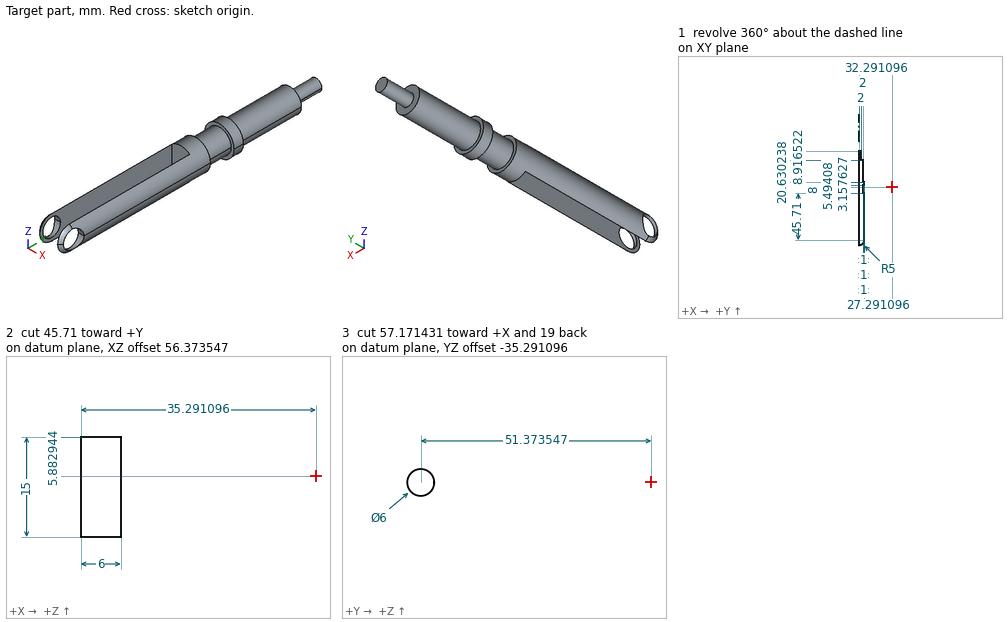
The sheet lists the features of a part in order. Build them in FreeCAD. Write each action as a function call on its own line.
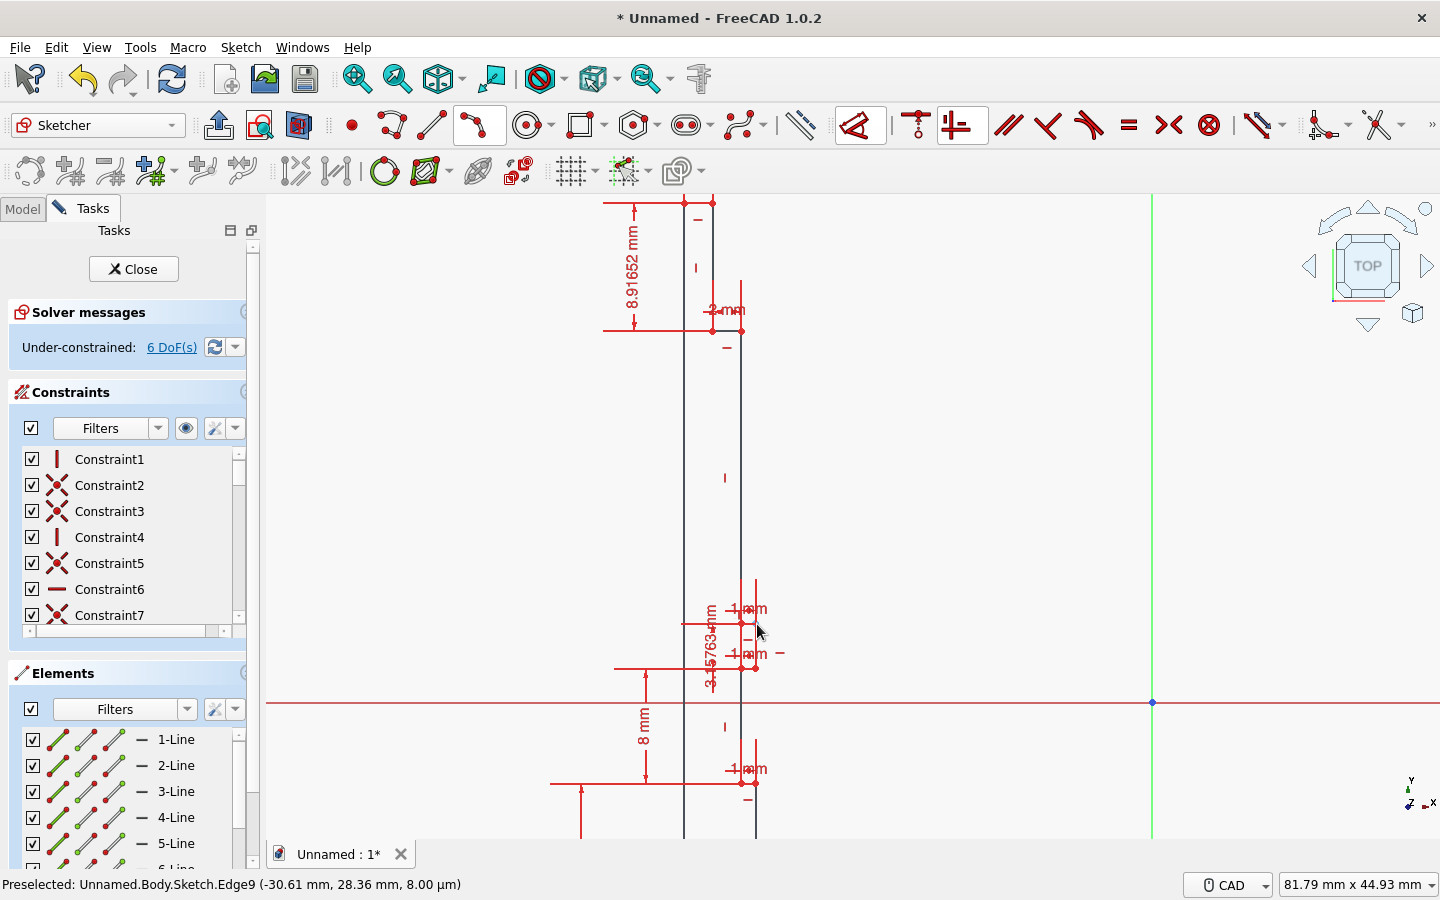
click(756, 624)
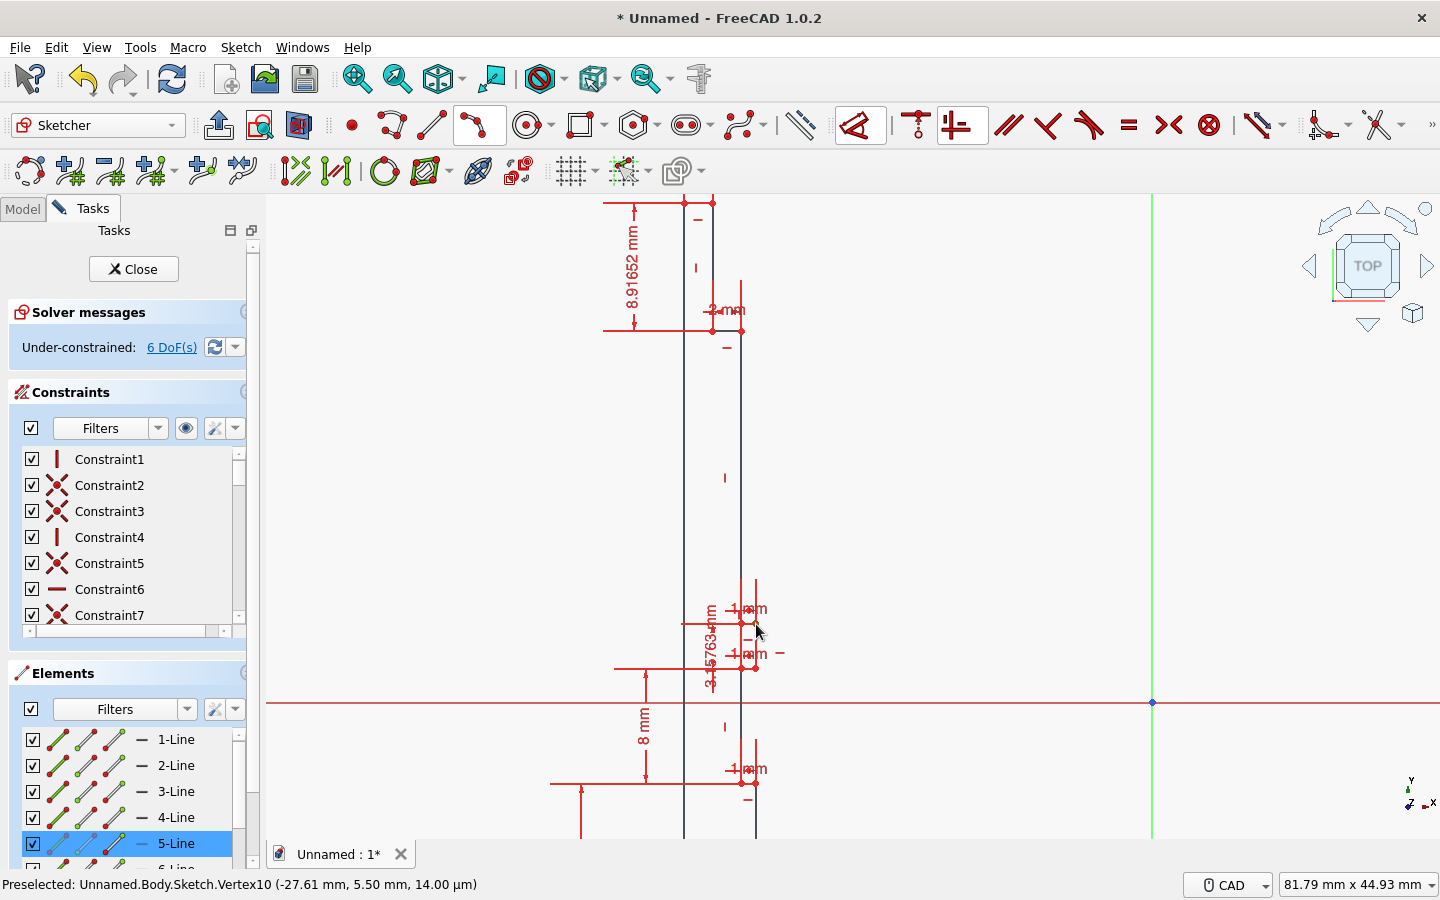
key(i)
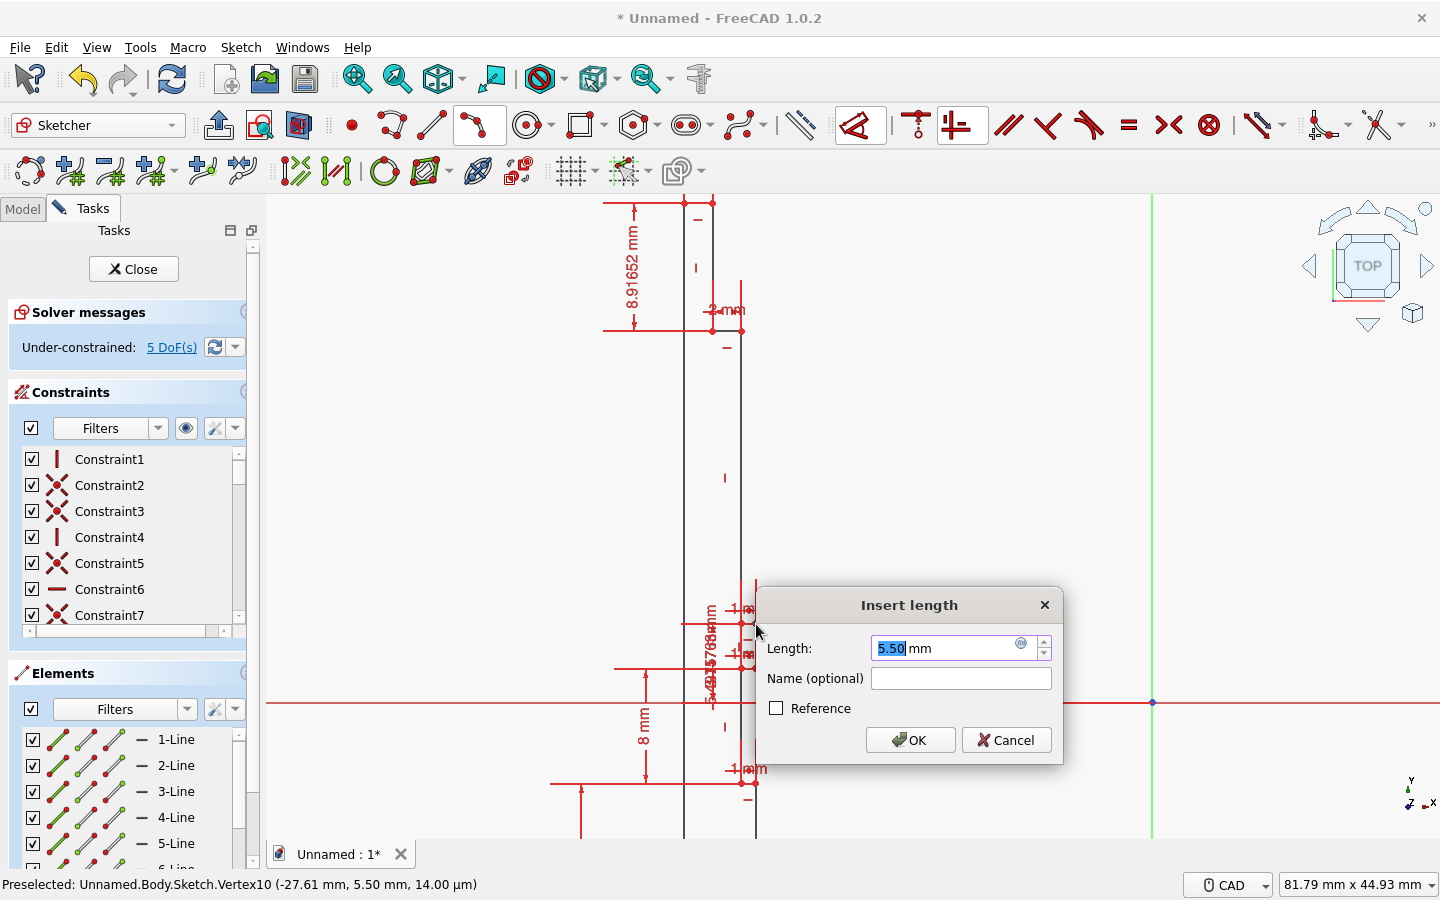
text(5.49408)
key(Return)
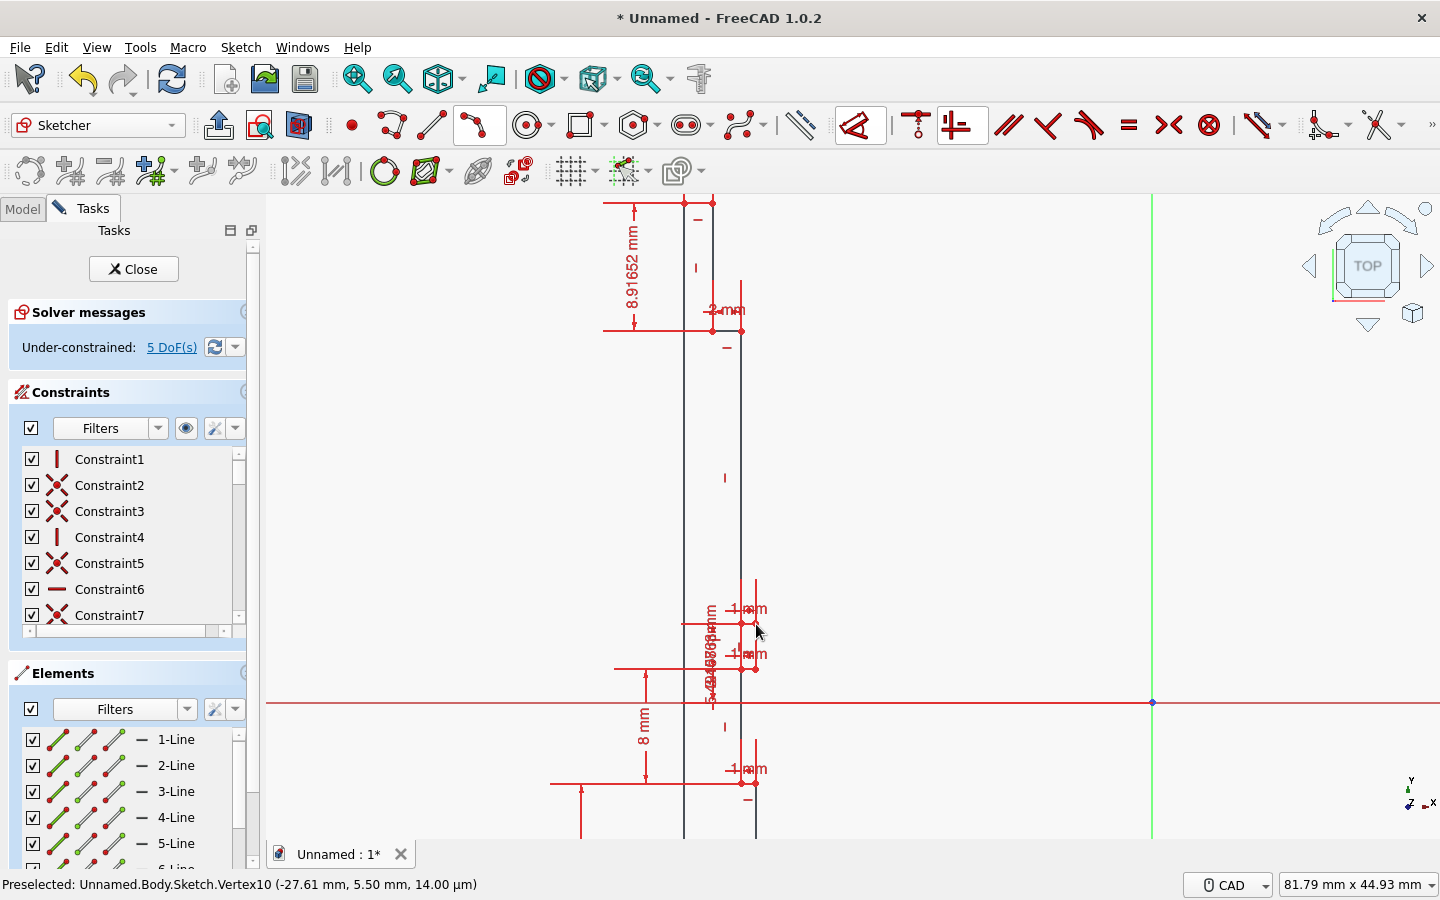
scroll(740, 491, down, 7)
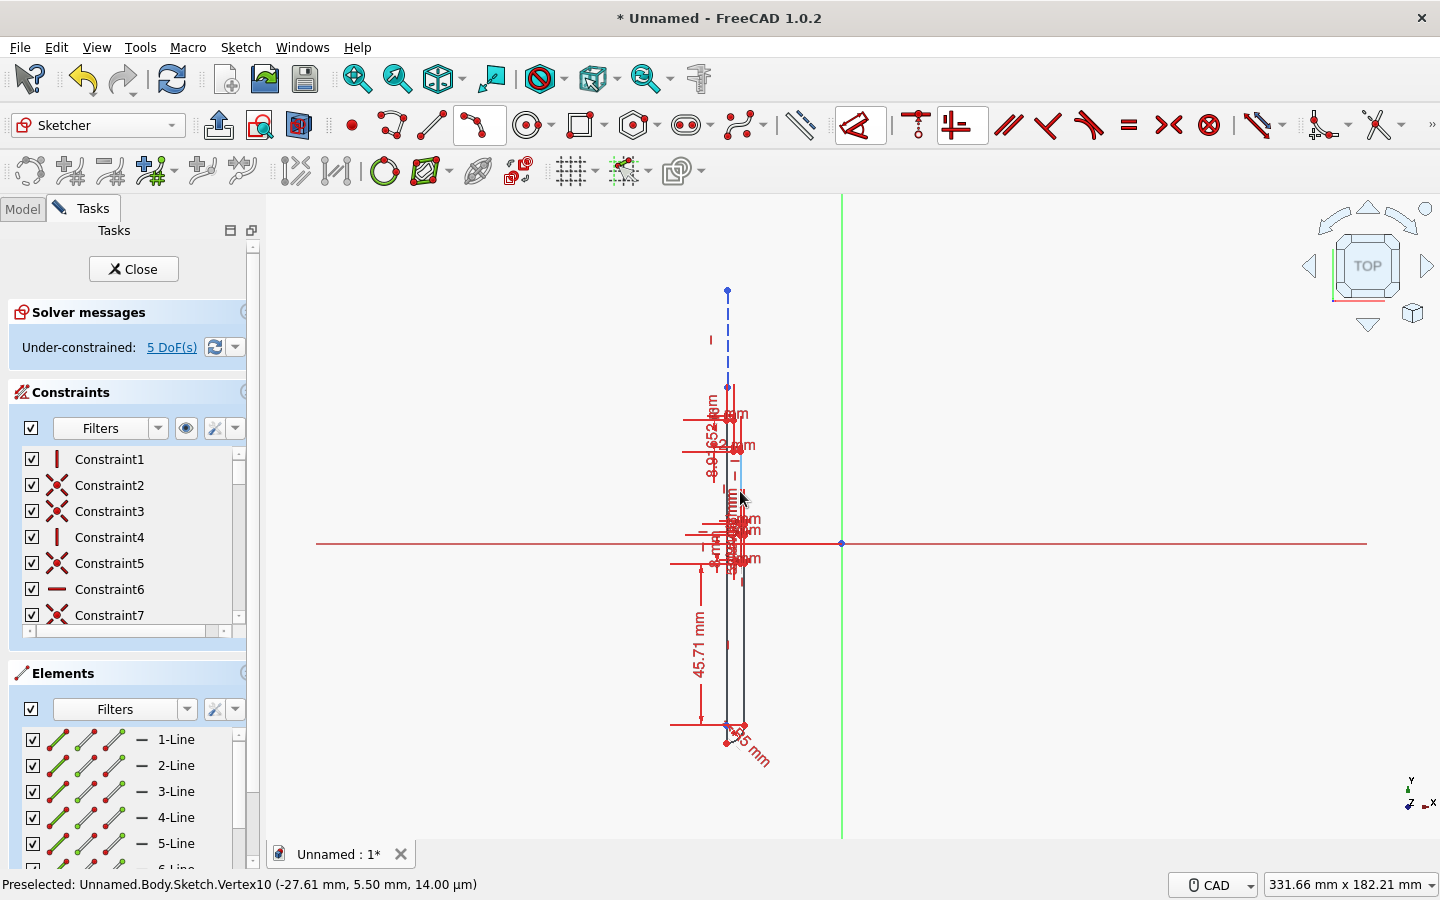
click(741, 481)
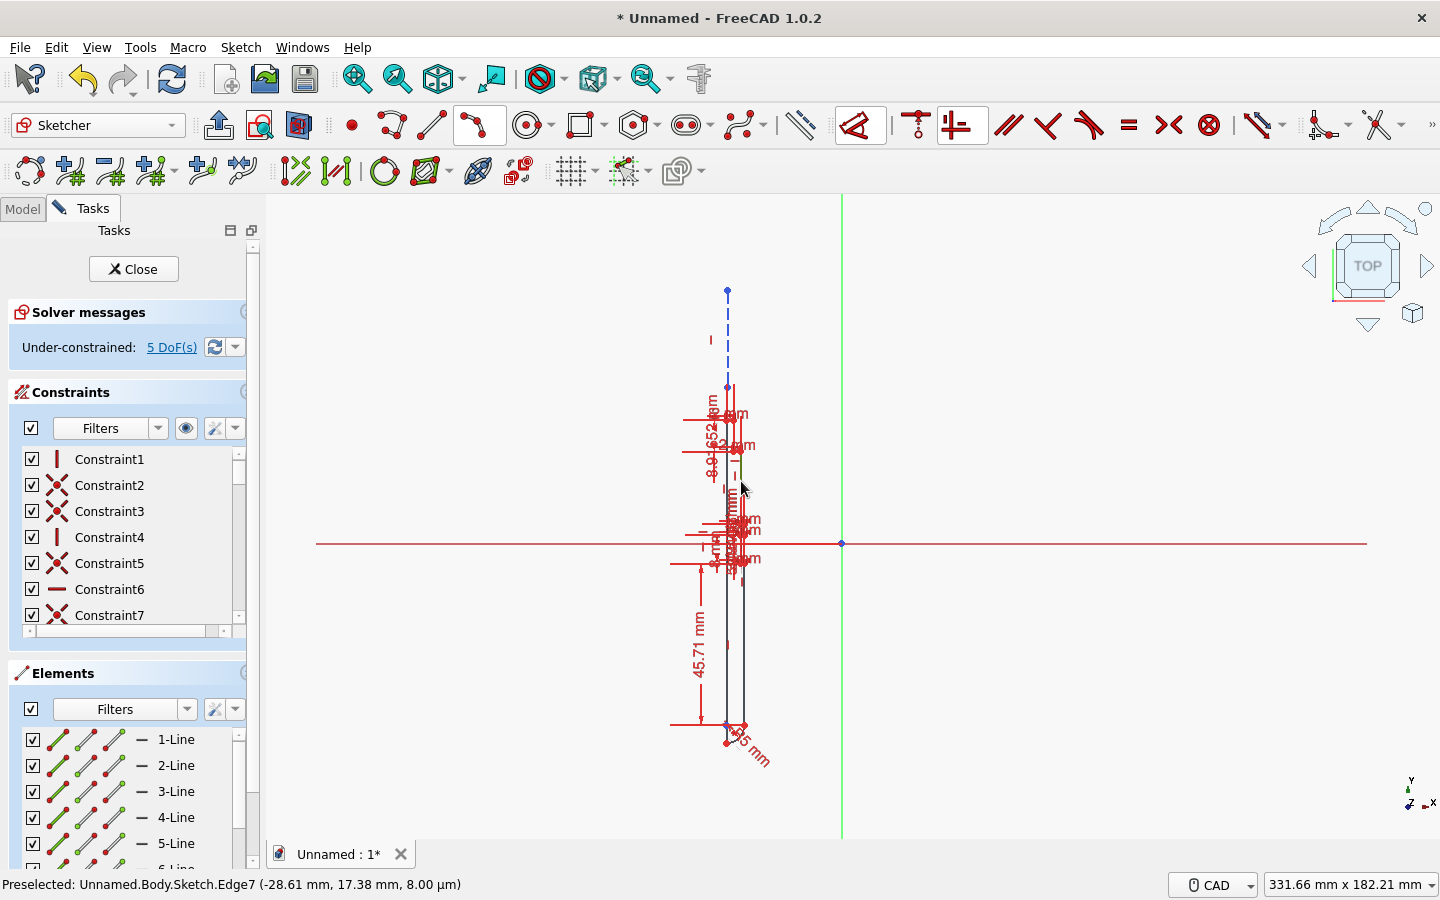
click(880, 126)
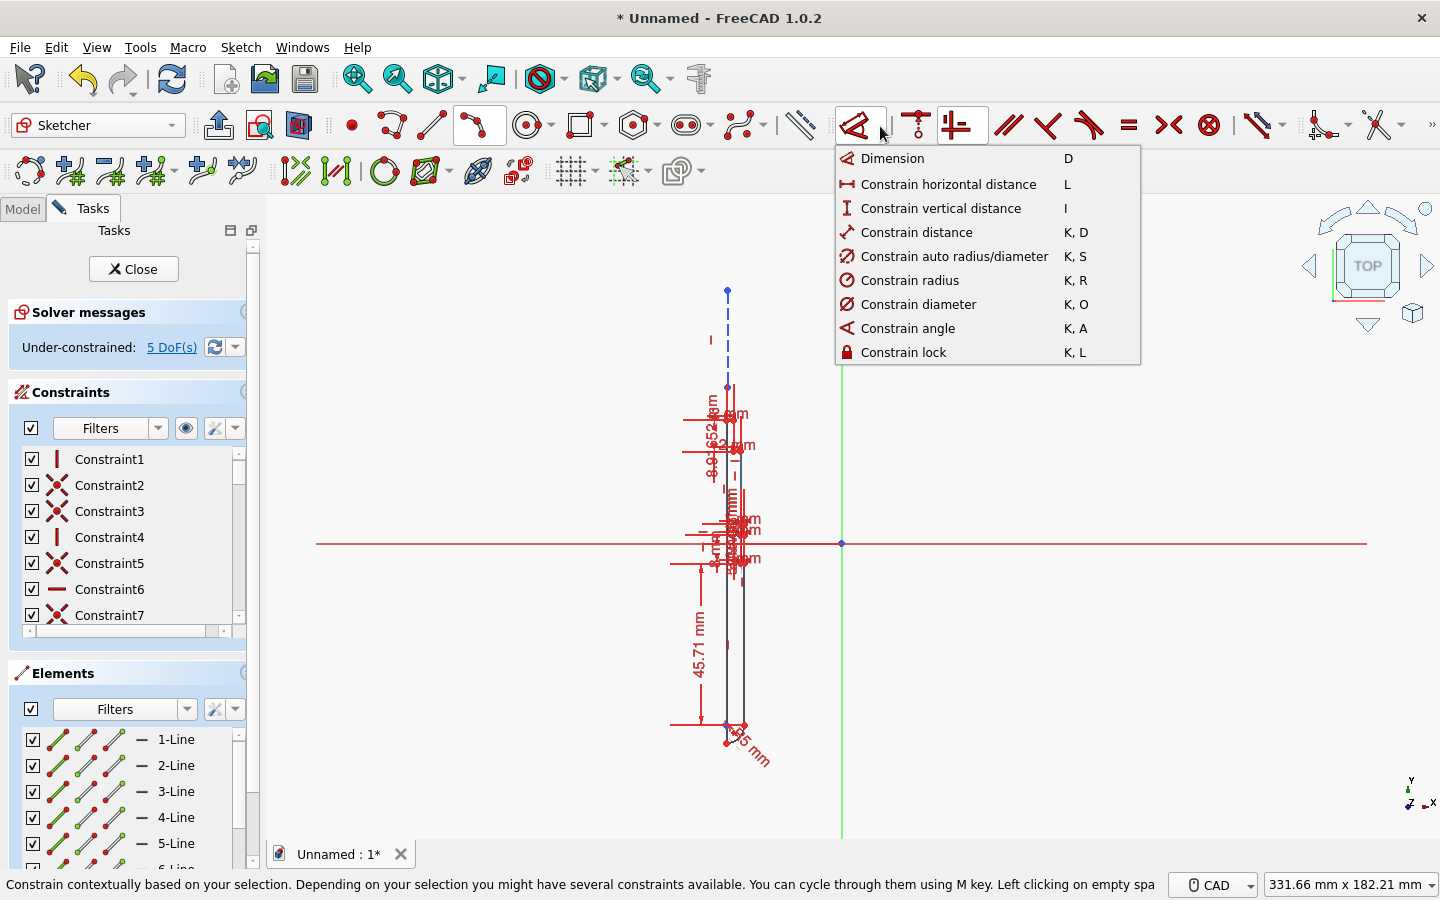
click(988, 208)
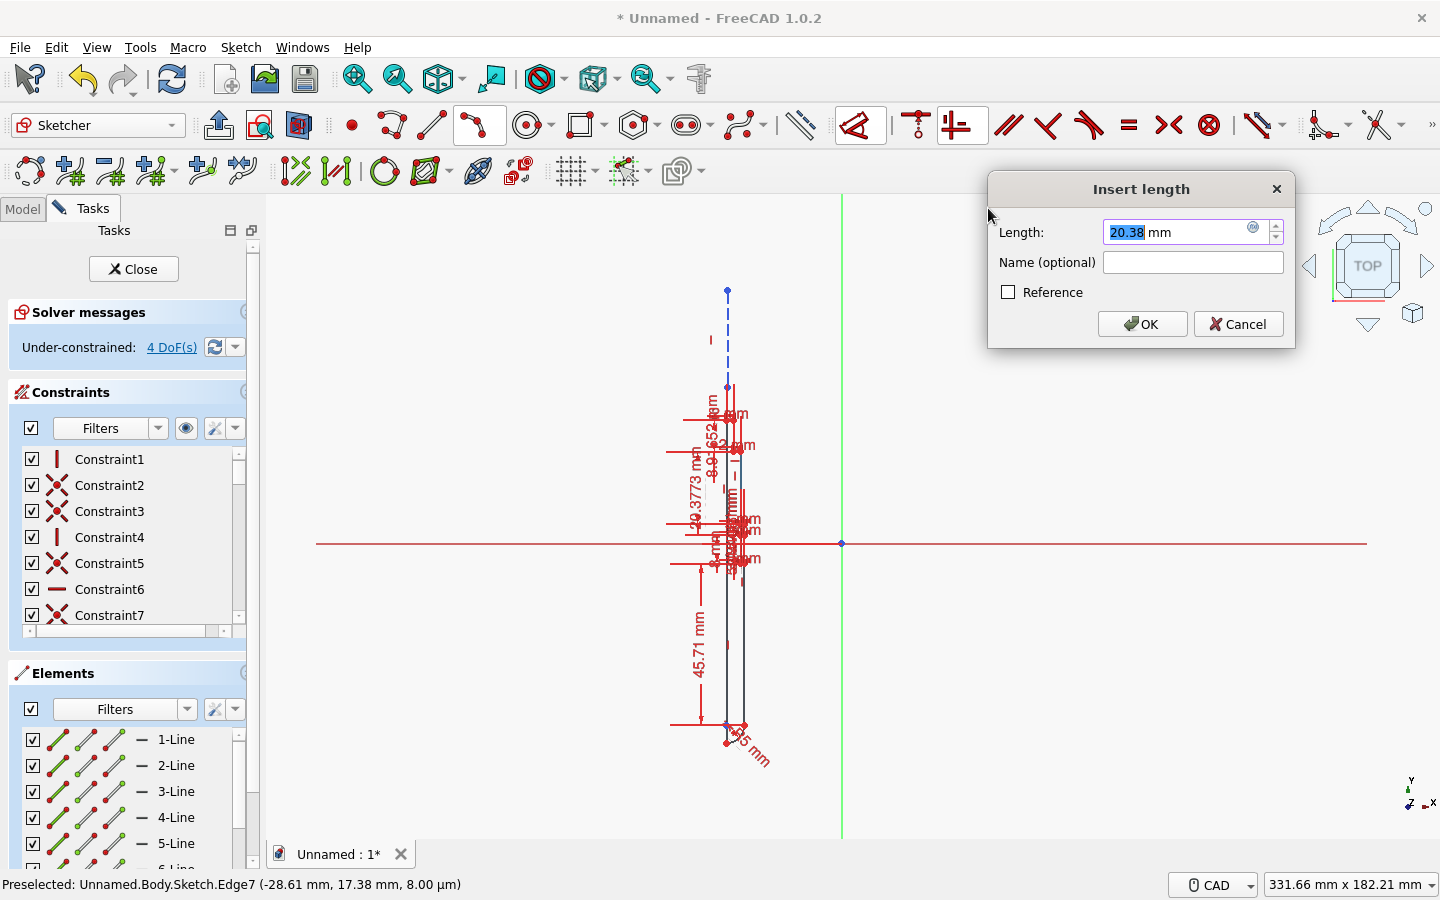
text(20.630238)
key(Return)